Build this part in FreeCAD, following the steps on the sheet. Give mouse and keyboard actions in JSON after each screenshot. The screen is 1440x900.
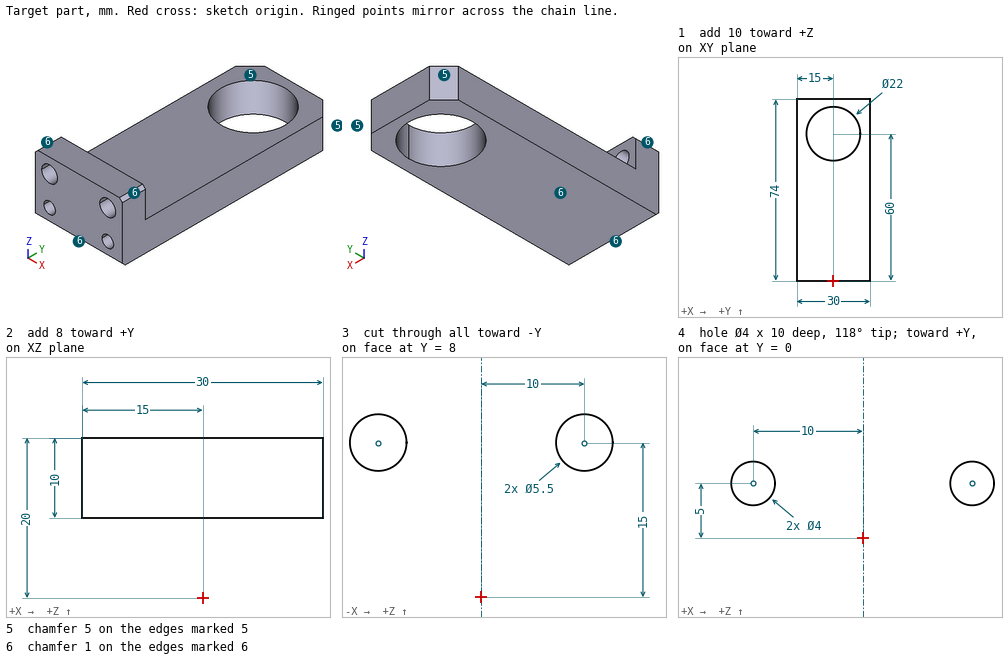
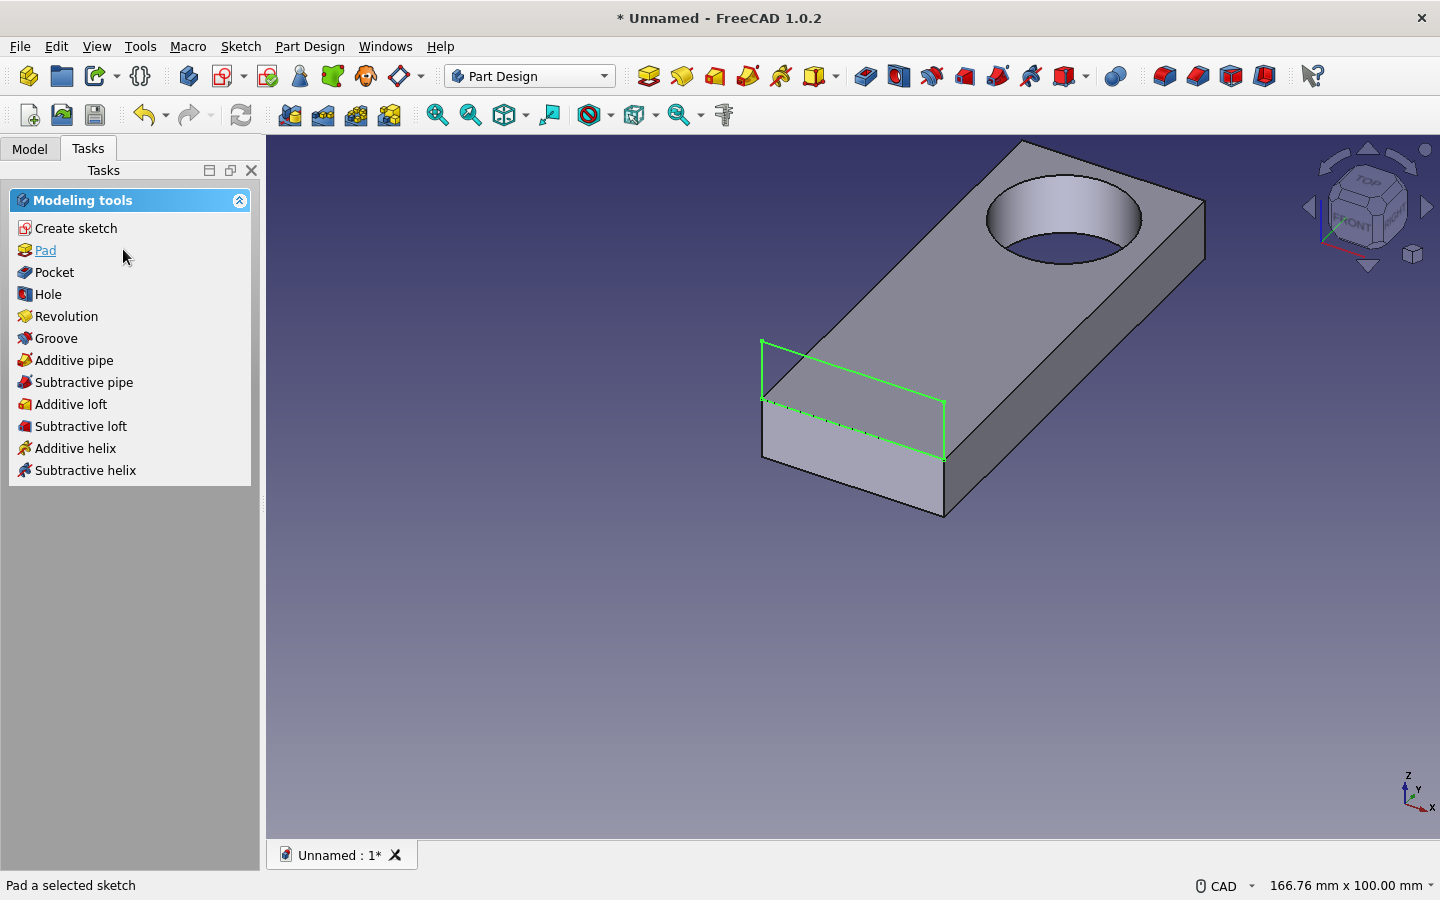
{"action": "left_click", "coordinate": [649, 76]}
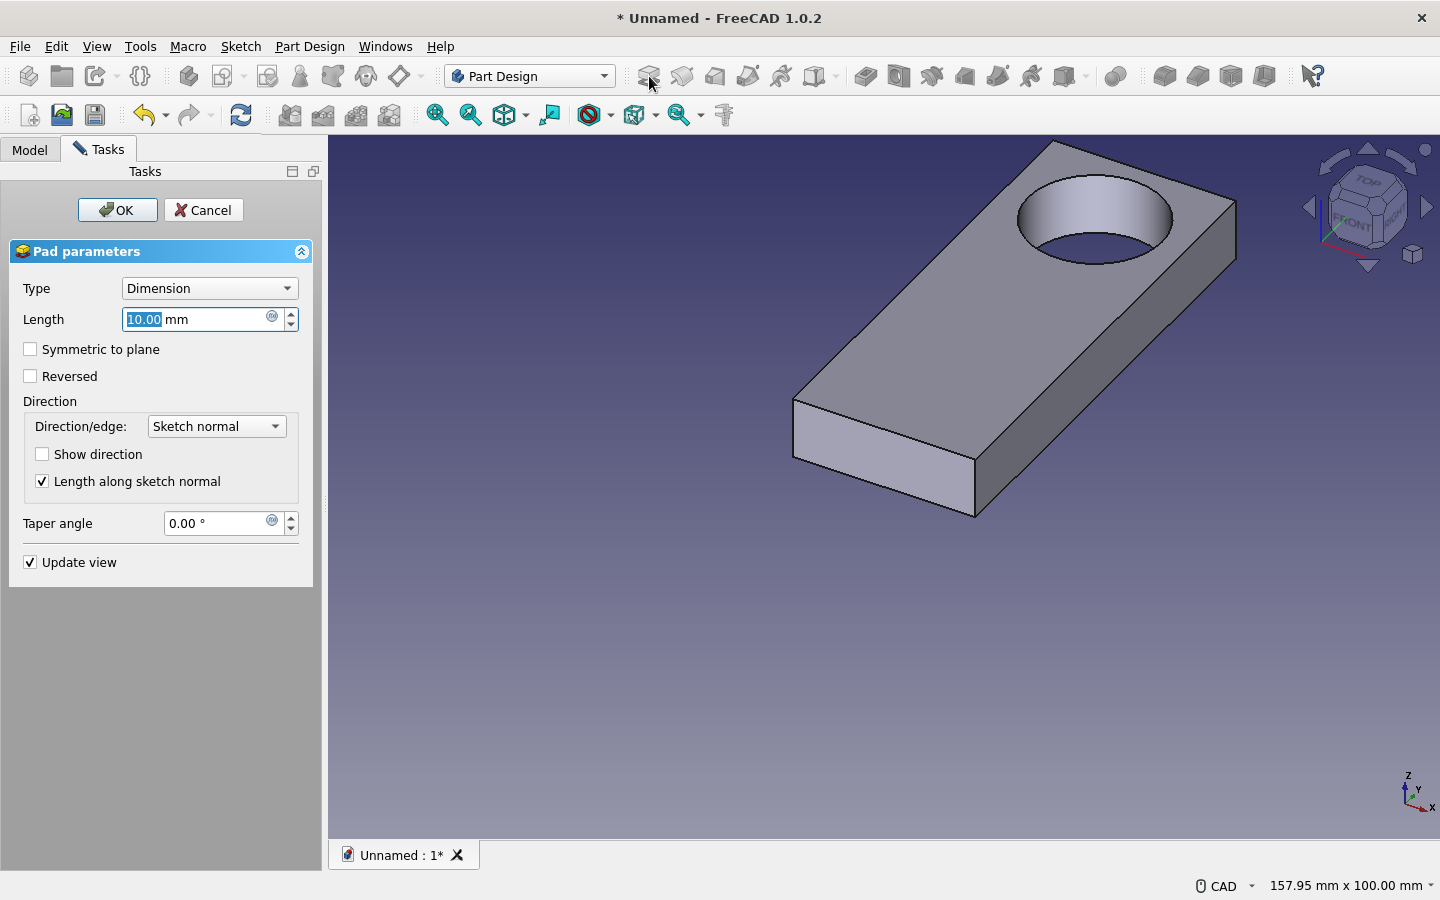
{"action": "type", "text": "8"}
{"action": "key", "text": "Tab"}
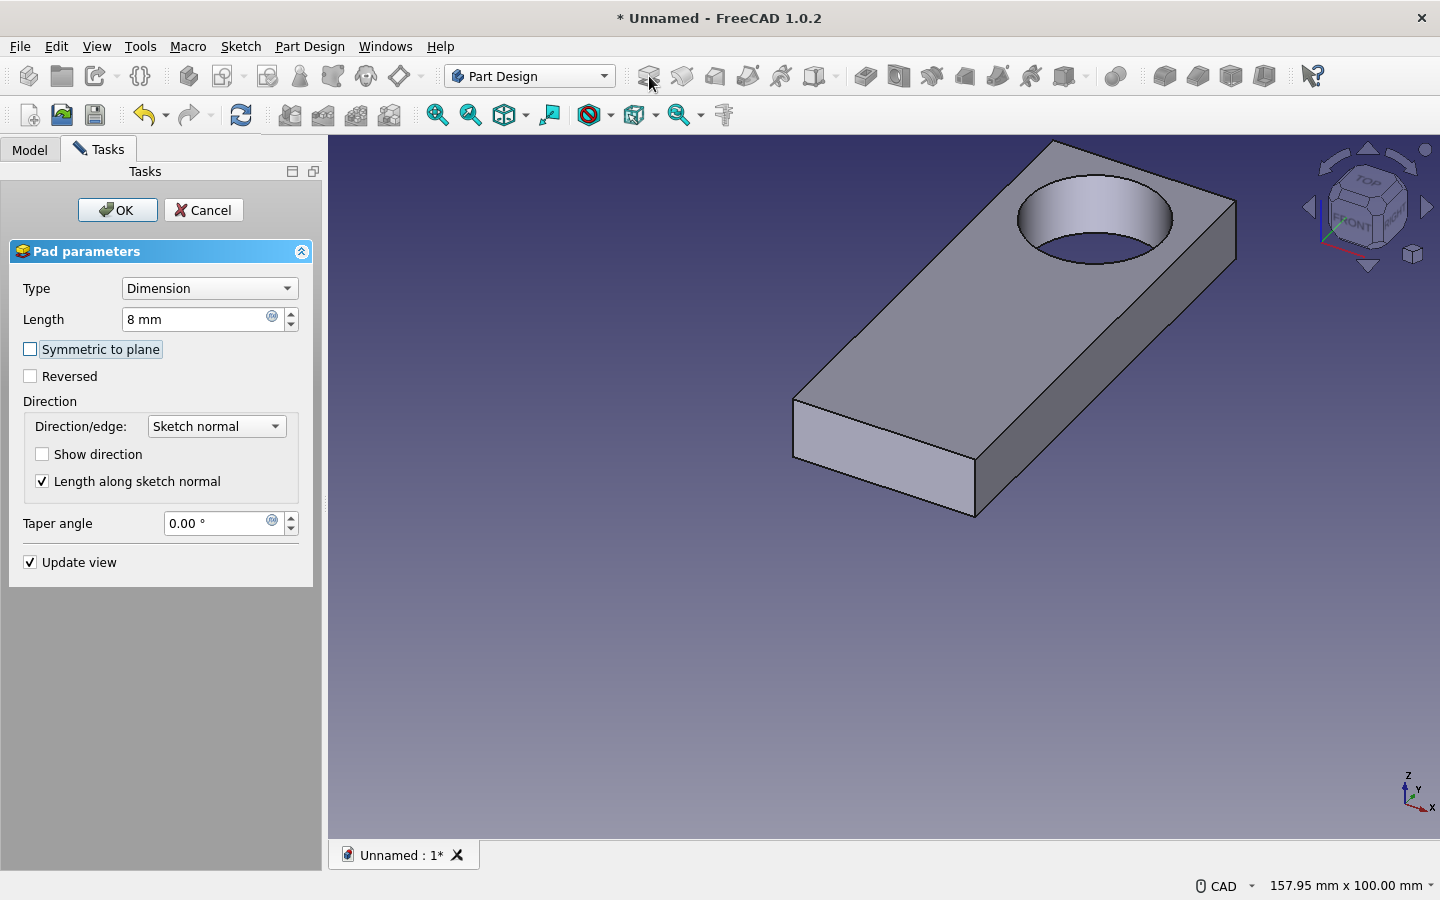
{"action": "left_click", "coordinate": [31, 376]}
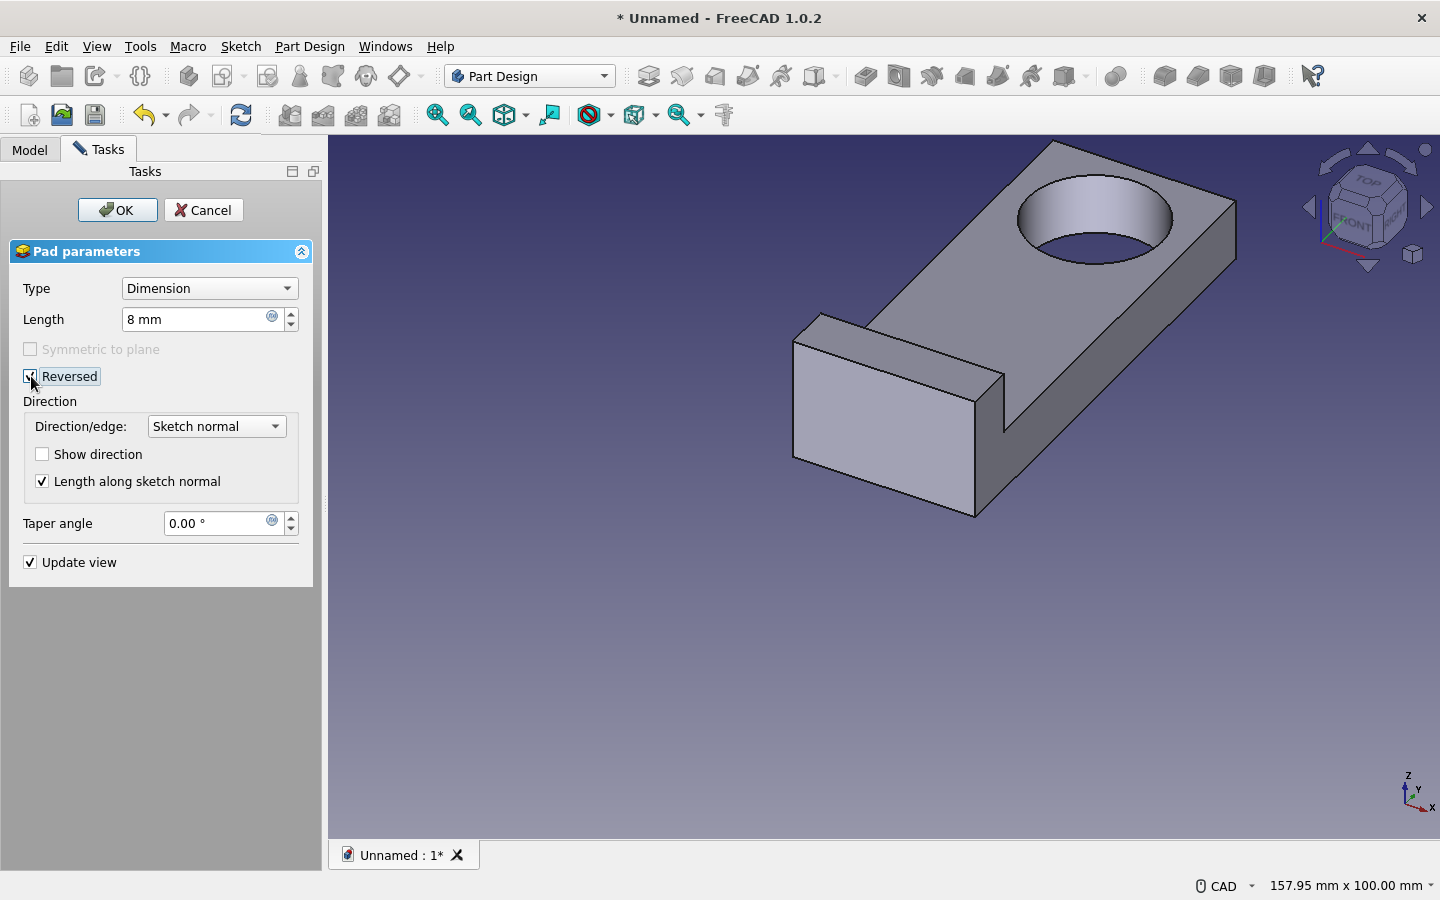
{"action": "left_click", "coordinate": [118, 210]}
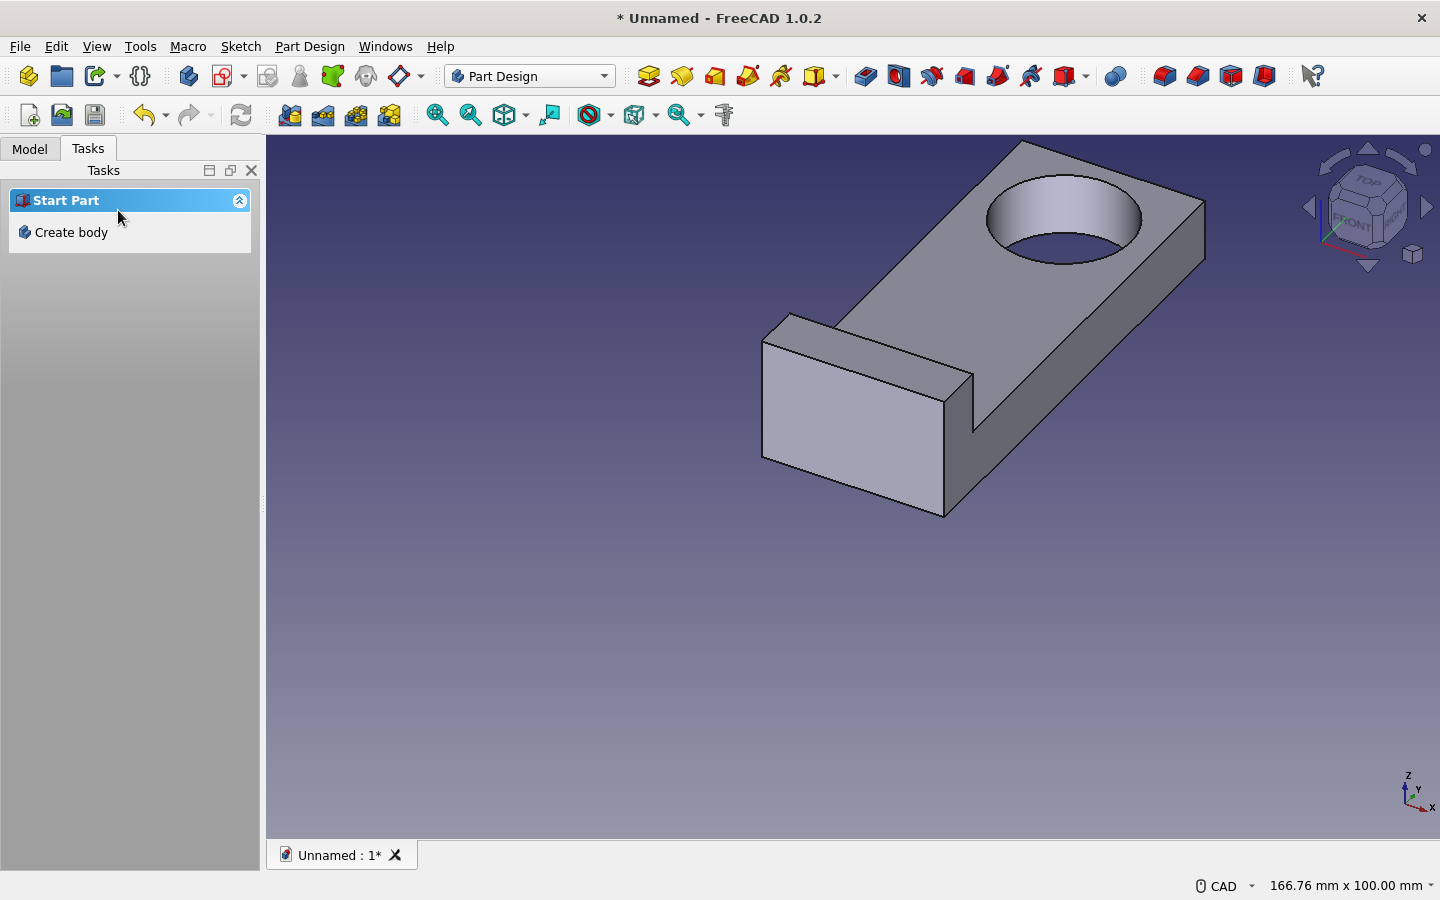
{"action": "left_click", "coordinate": [438, 116]}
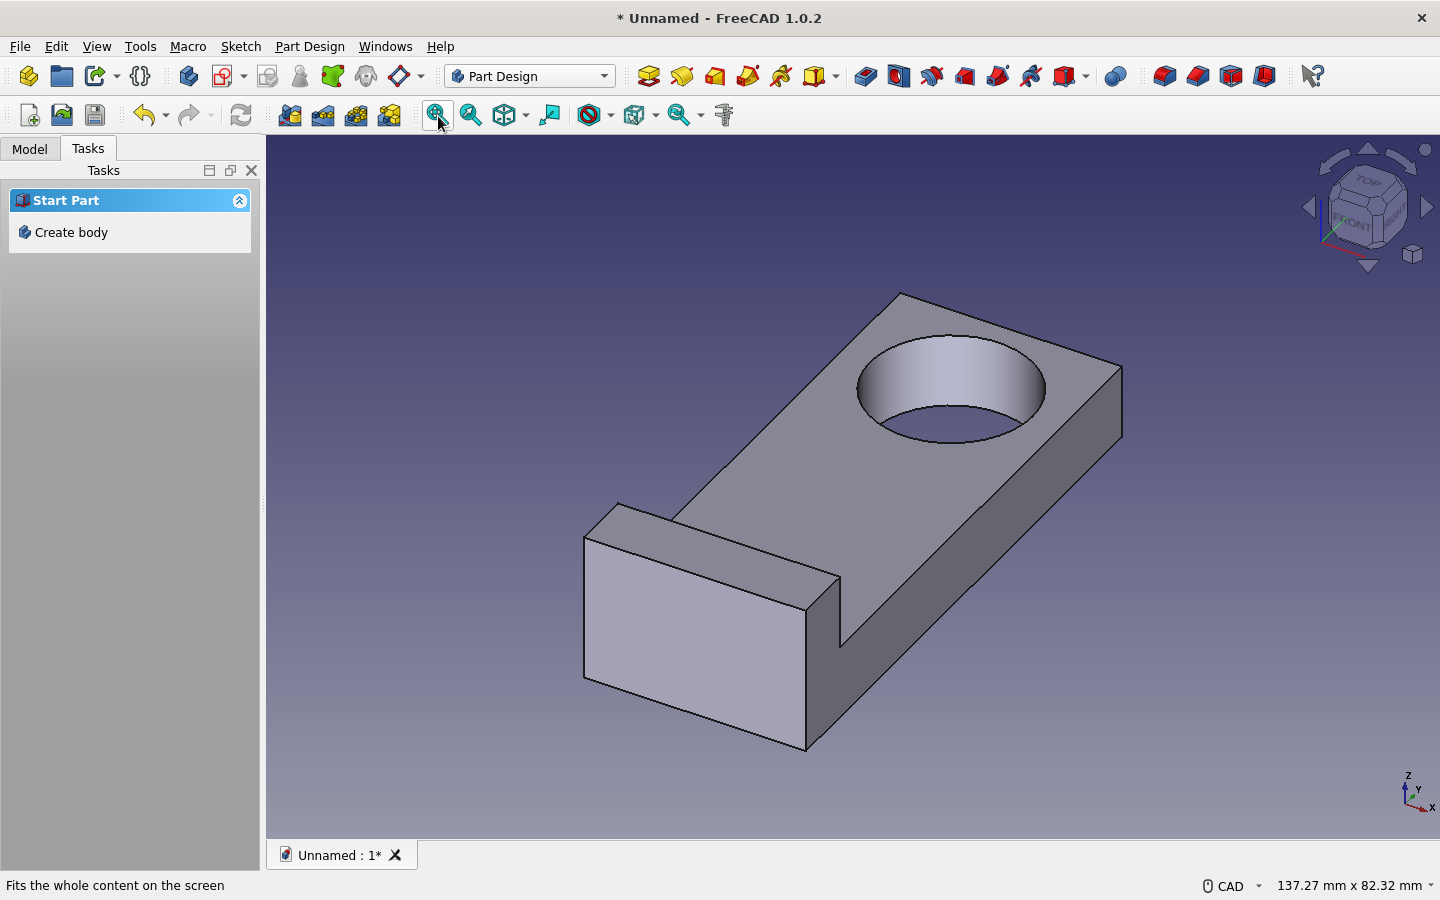
{"action": "key", "text": "4"}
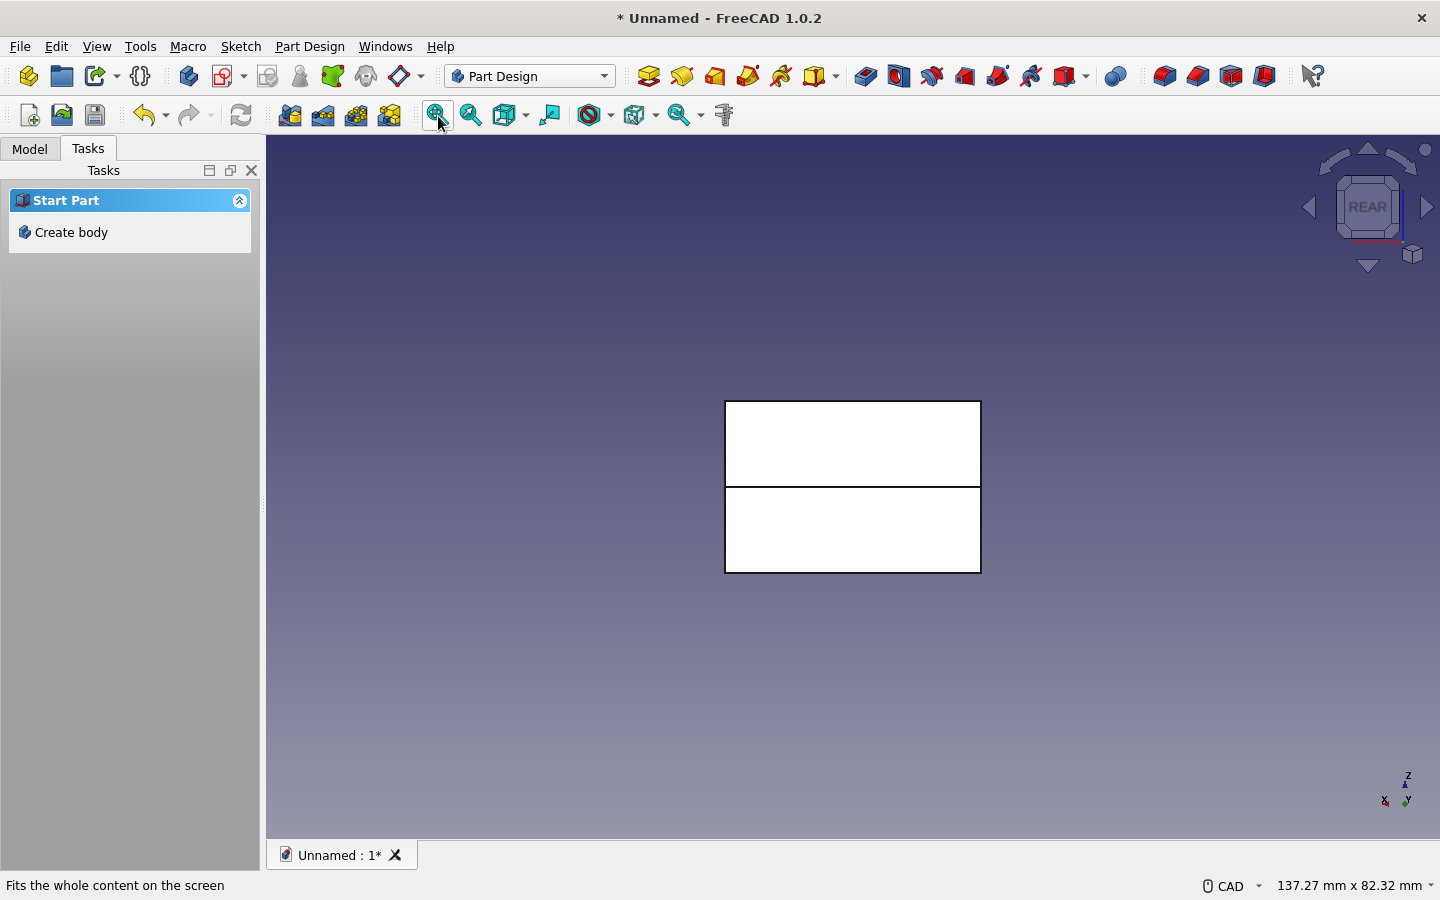
{"action": "left_click", "coordinate": [438, 116]}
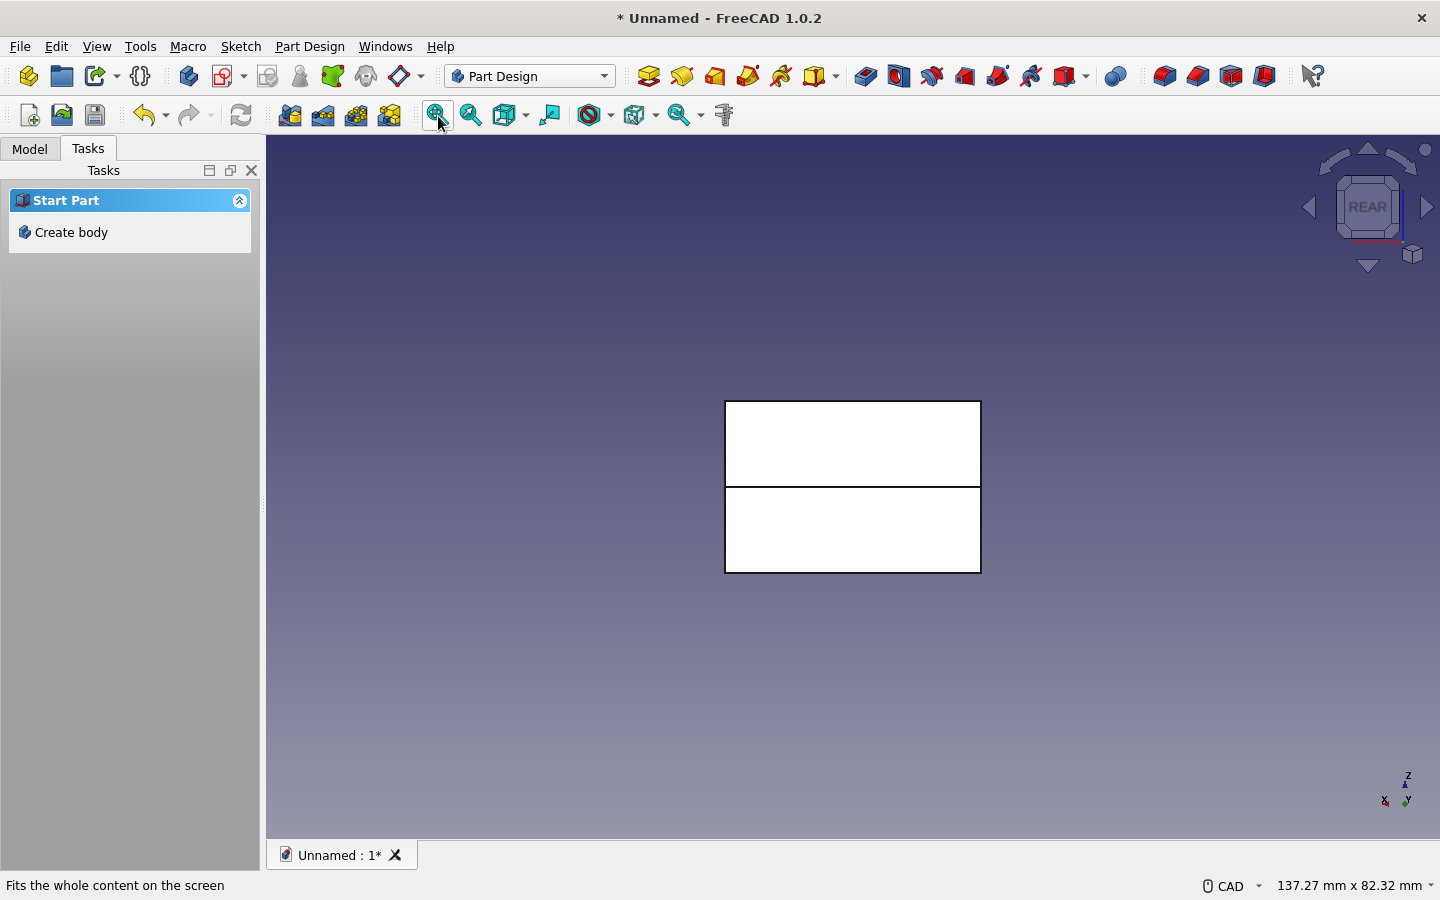
{"action": "left_click", "coordinate": [780, 443]}